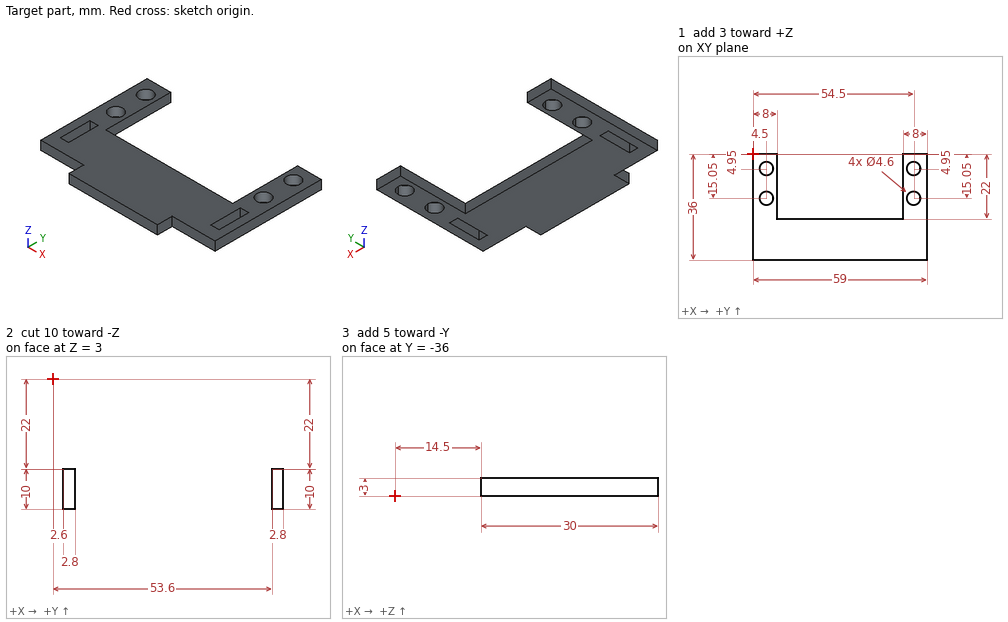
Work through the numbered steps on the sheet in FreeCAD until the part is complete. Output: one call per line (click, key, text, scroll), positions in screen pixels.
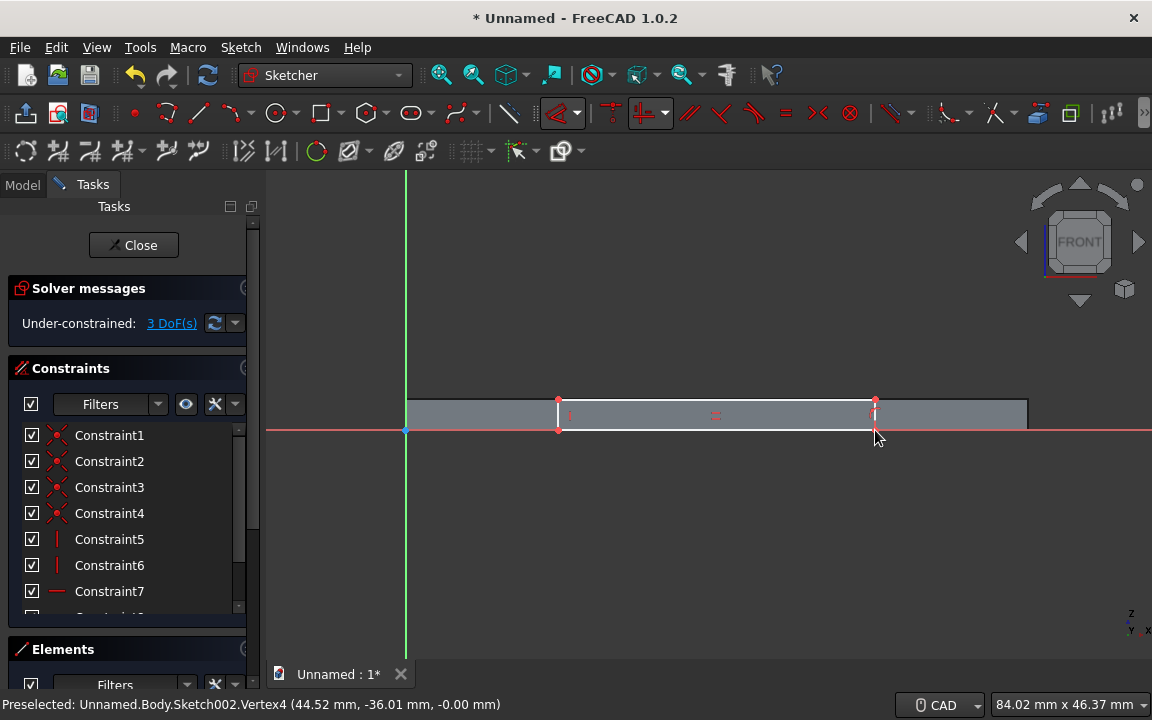
click(556, 114)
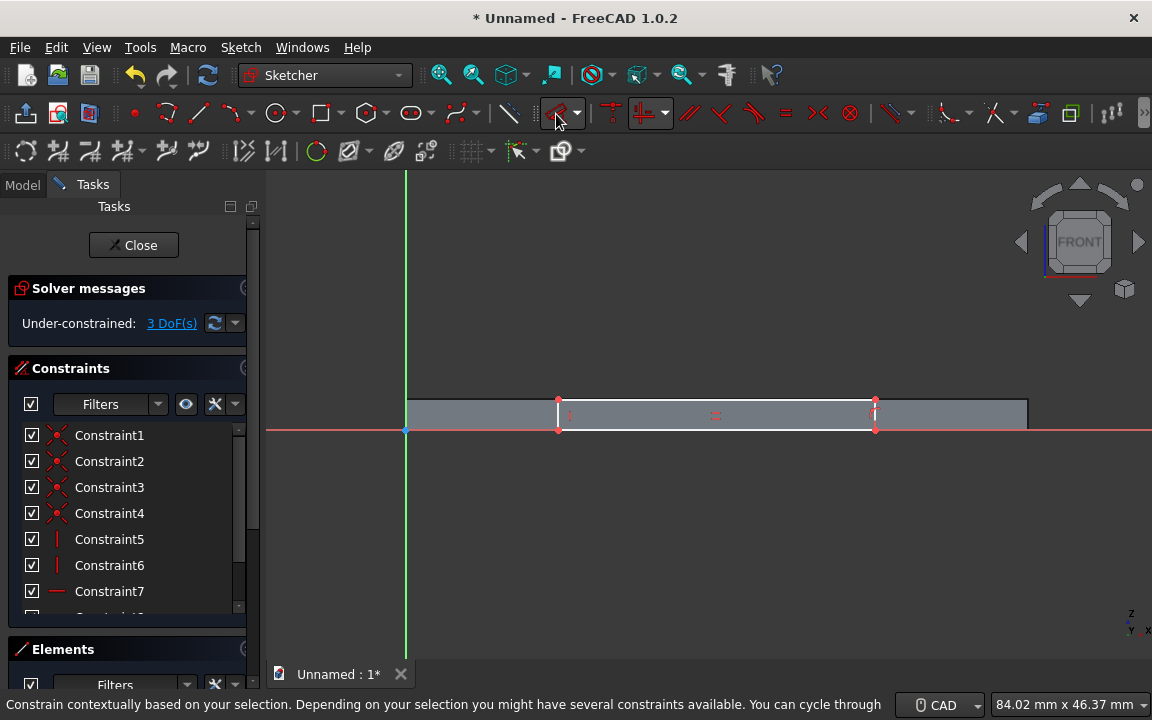
scroll(558, 409, up, 3)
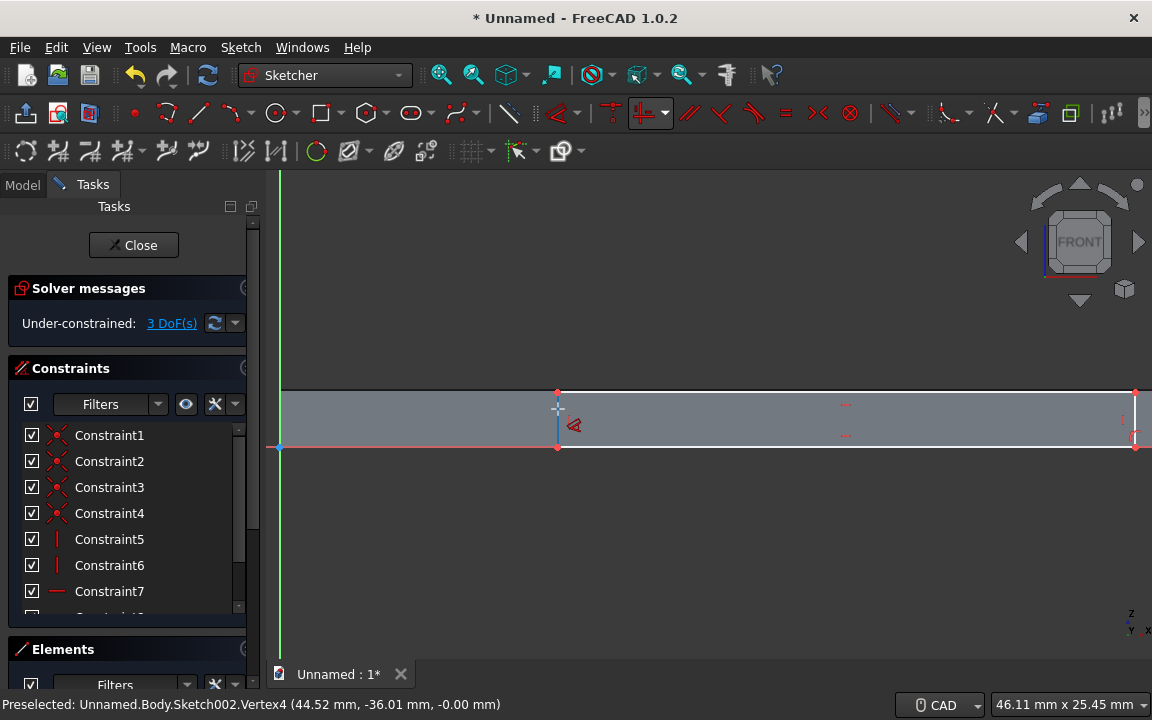
click(558, 409)
click(524, 420)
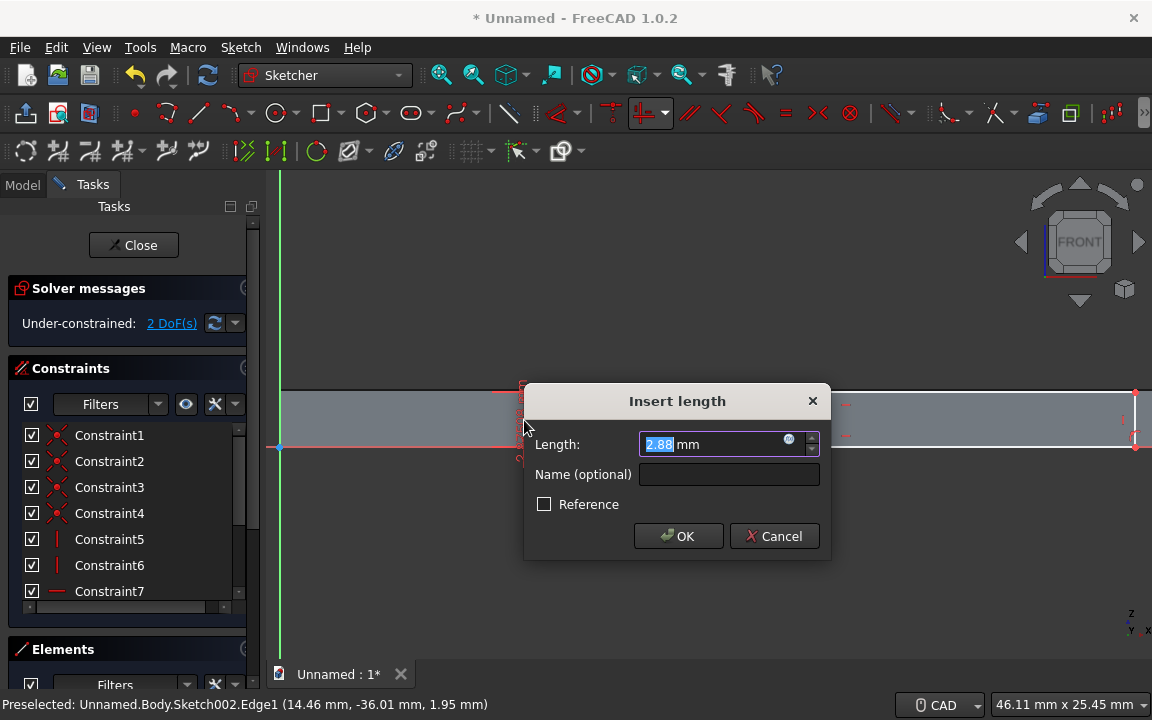
text(3)
key(Return)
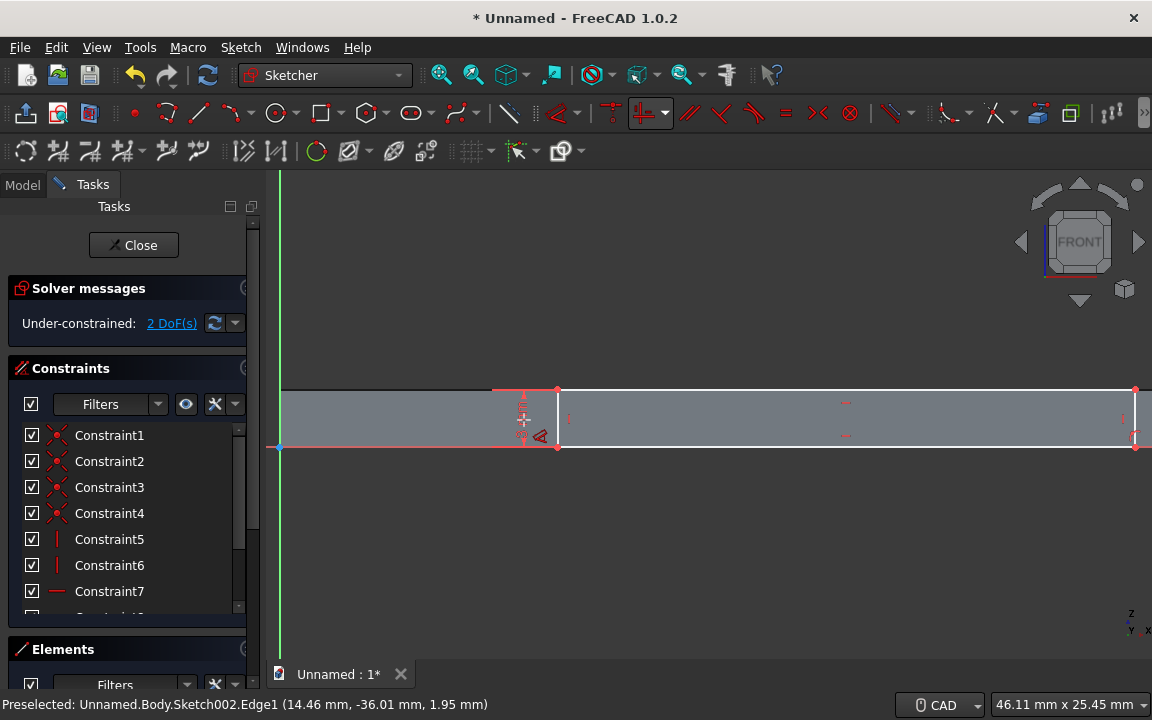
click(731, 447)
click(772, 481)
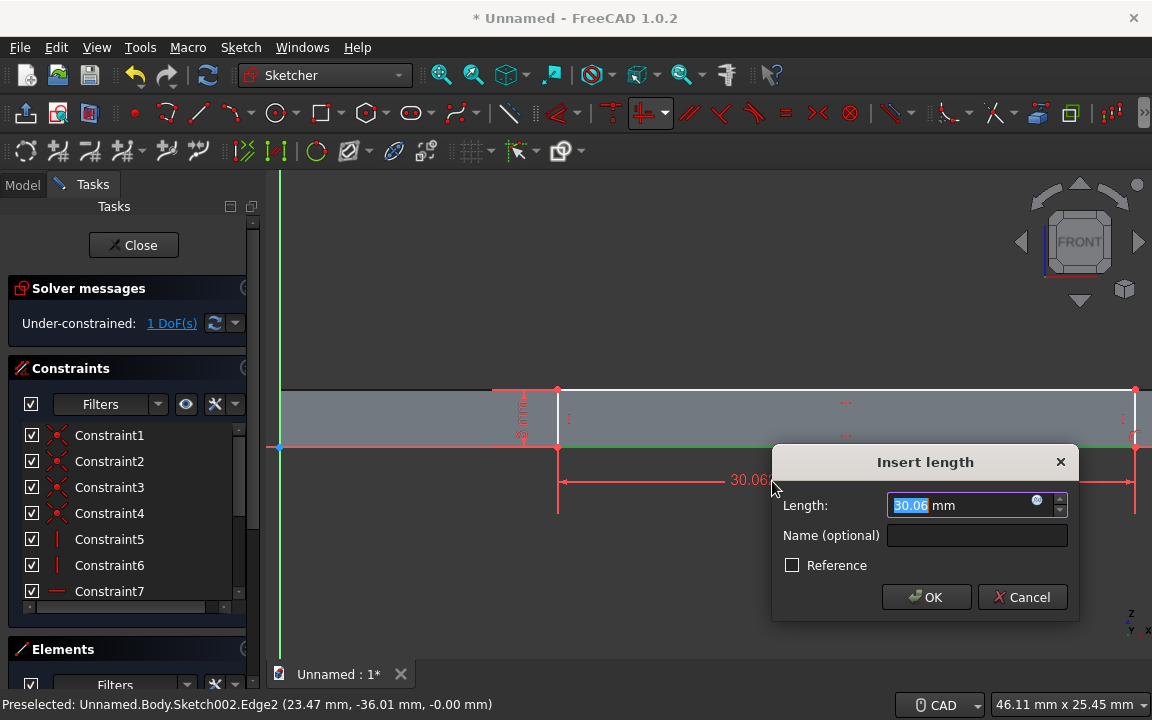
text(30)
key(Return)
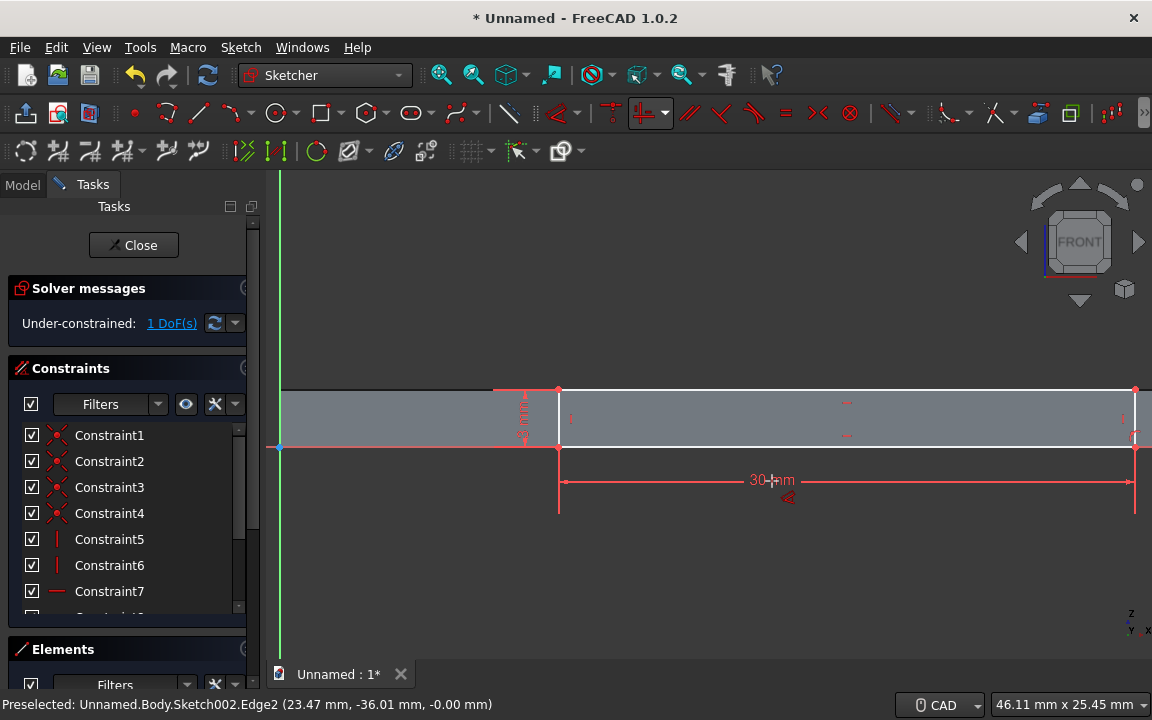
click(559, 390)
click(426, 481)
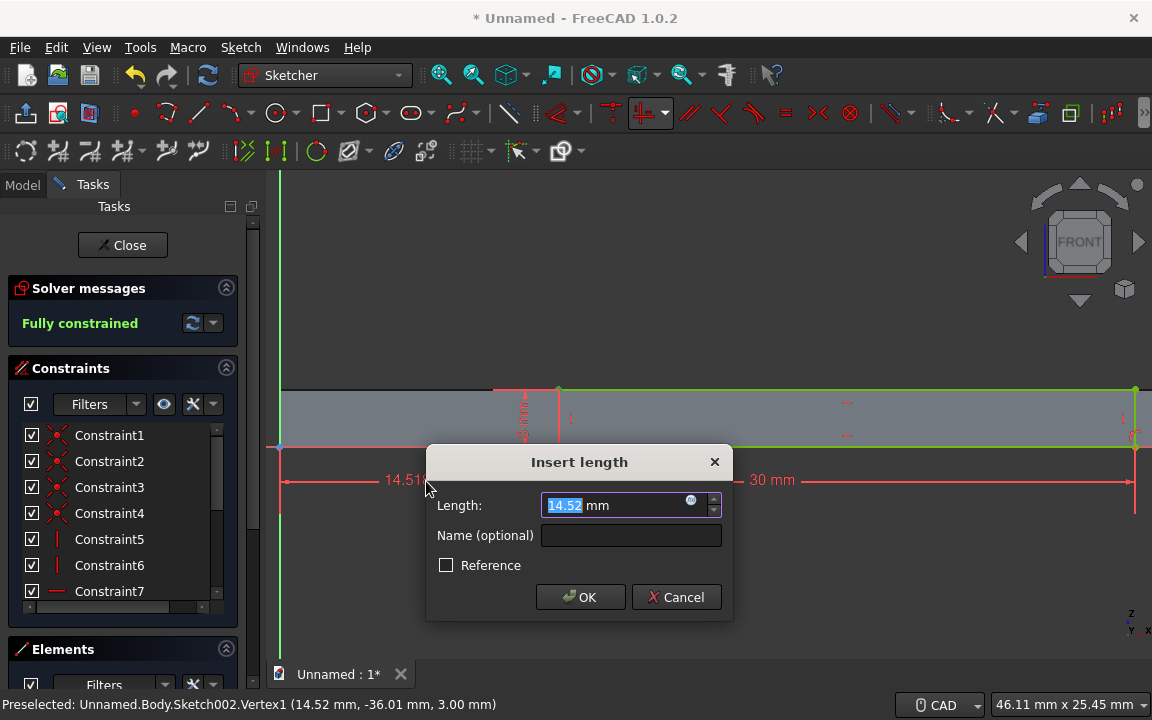
text(14.5)
key(Return)
key(Escape)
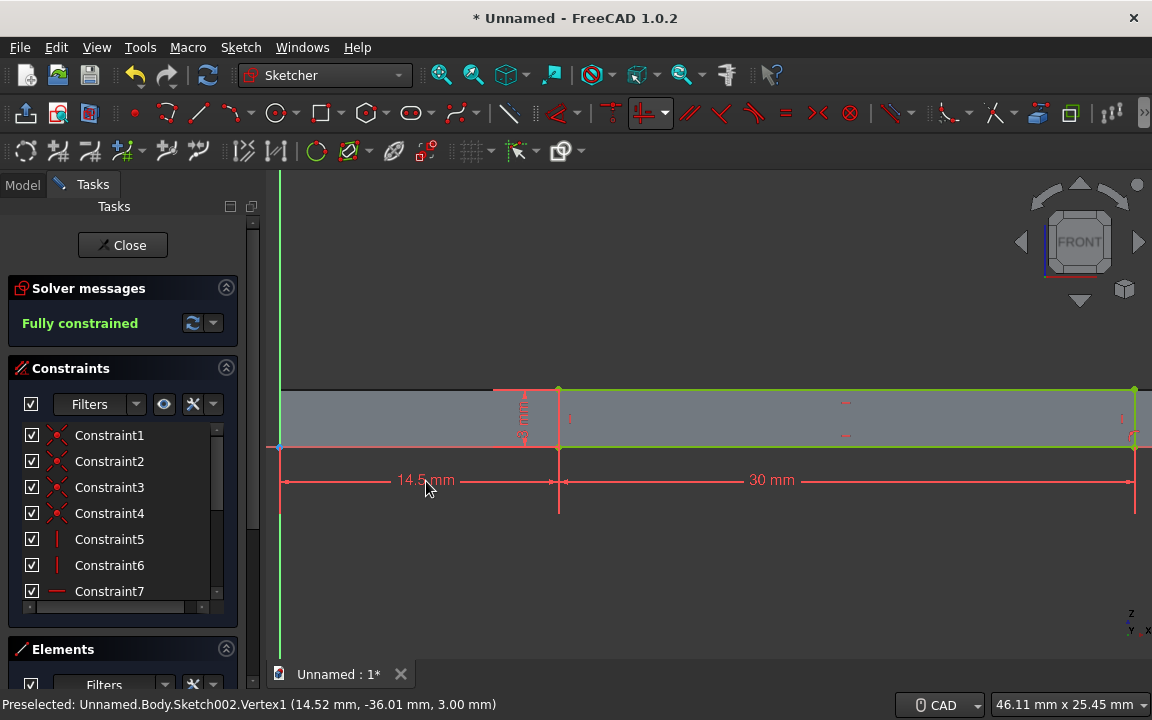
click(123, 245)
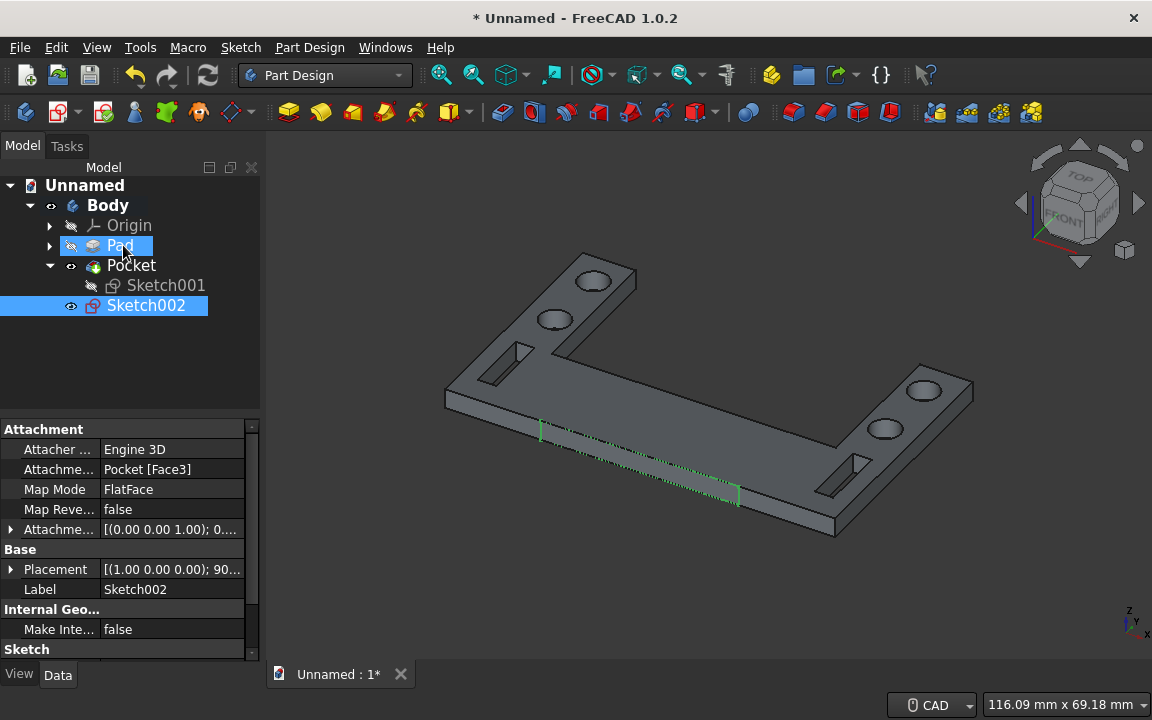
click(290, 112)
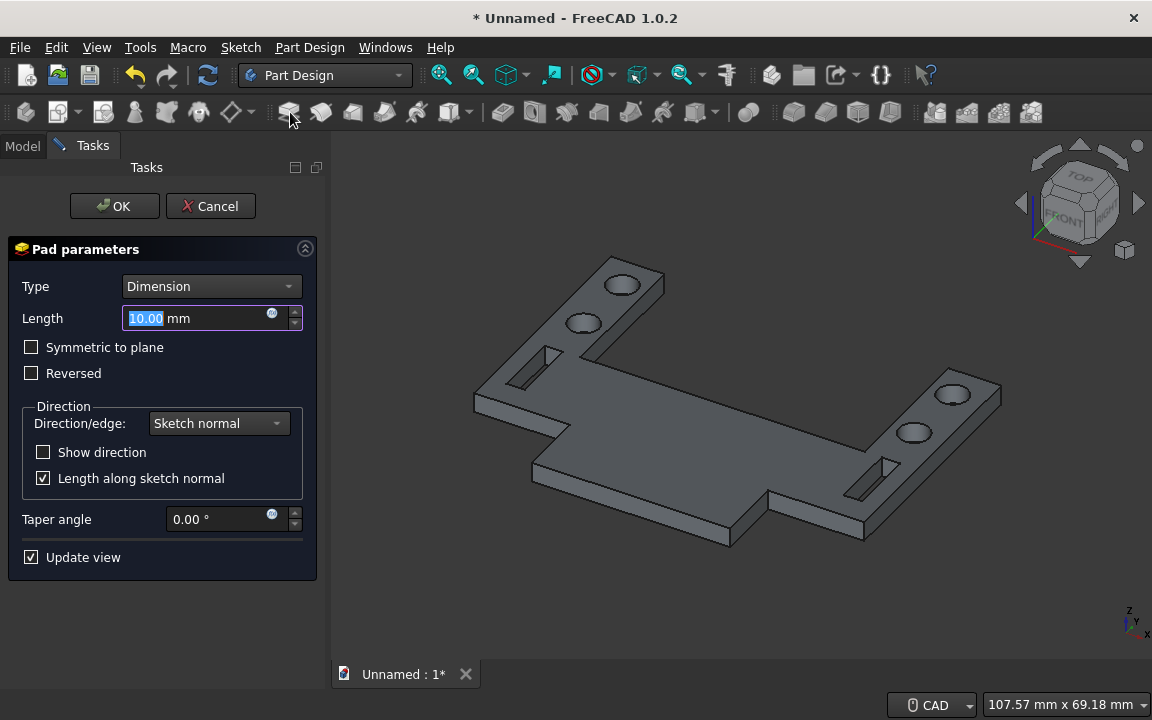
text(5)
key(Tab)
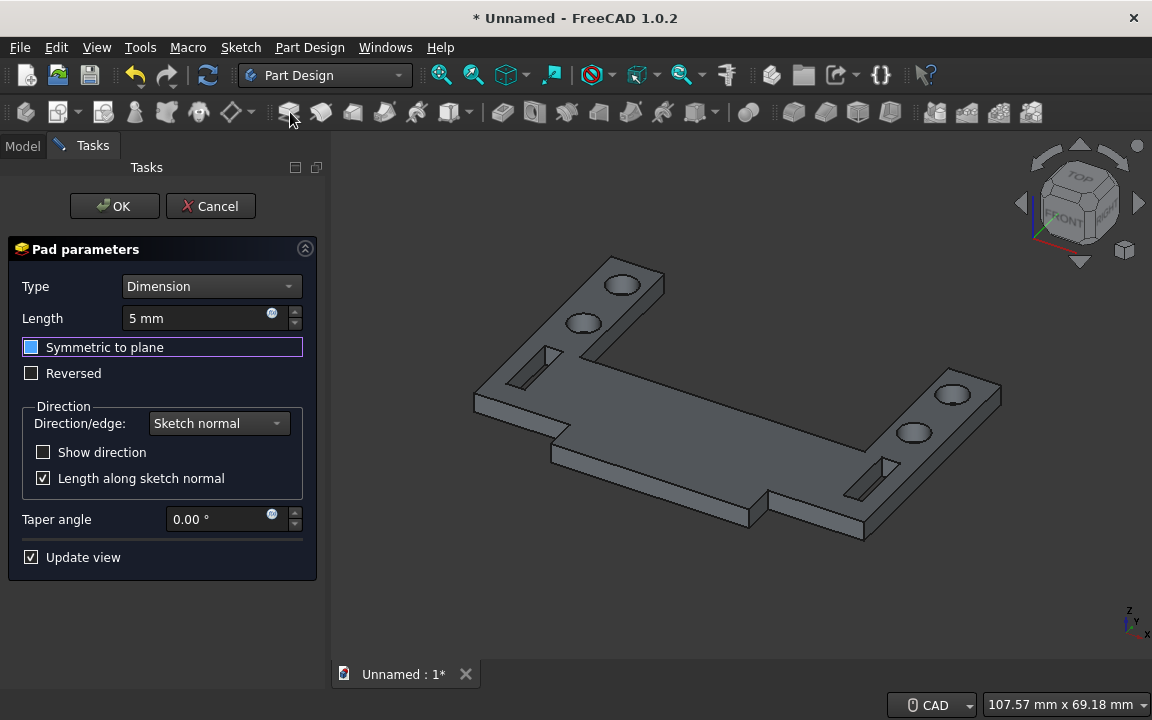
click(115, 206)